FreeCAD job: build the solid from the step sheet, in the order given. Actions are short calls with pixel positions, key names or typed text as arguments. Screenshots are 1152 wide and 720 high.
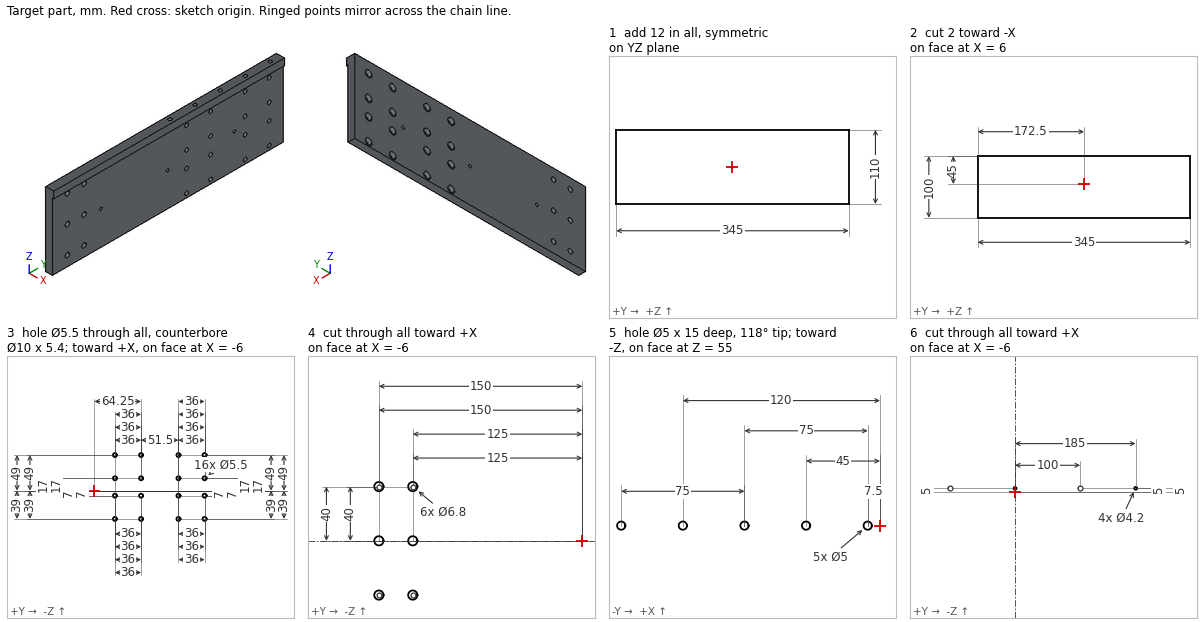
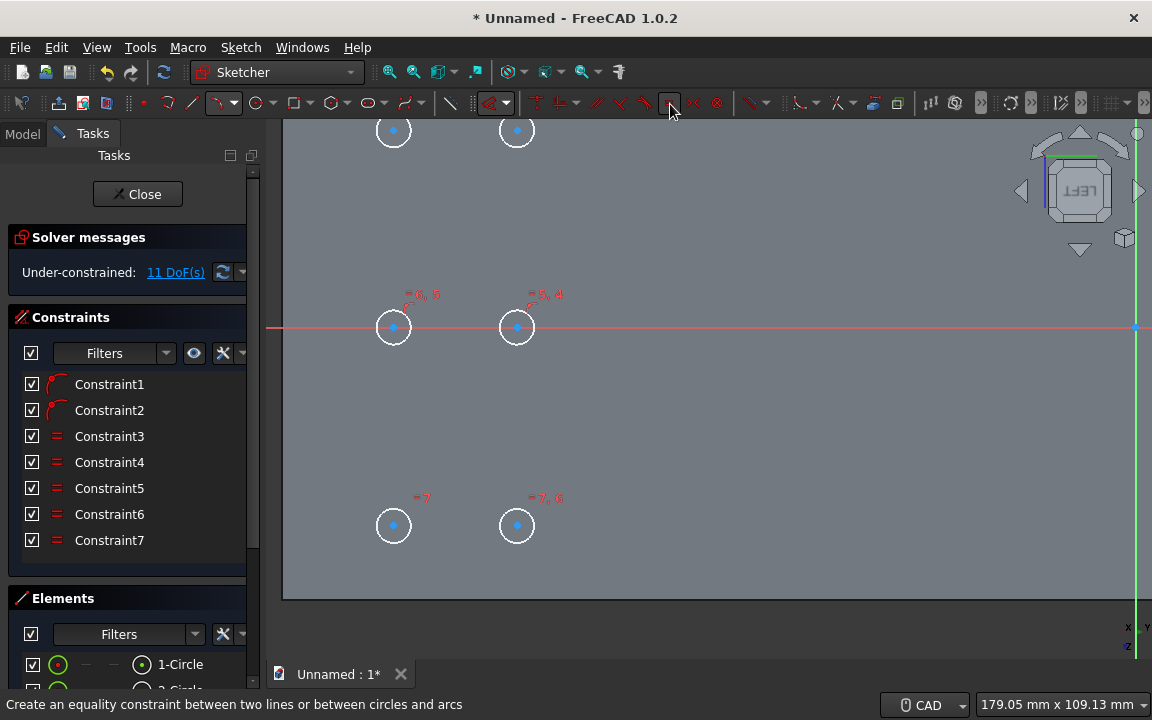
scroll(405, 514, down, 2)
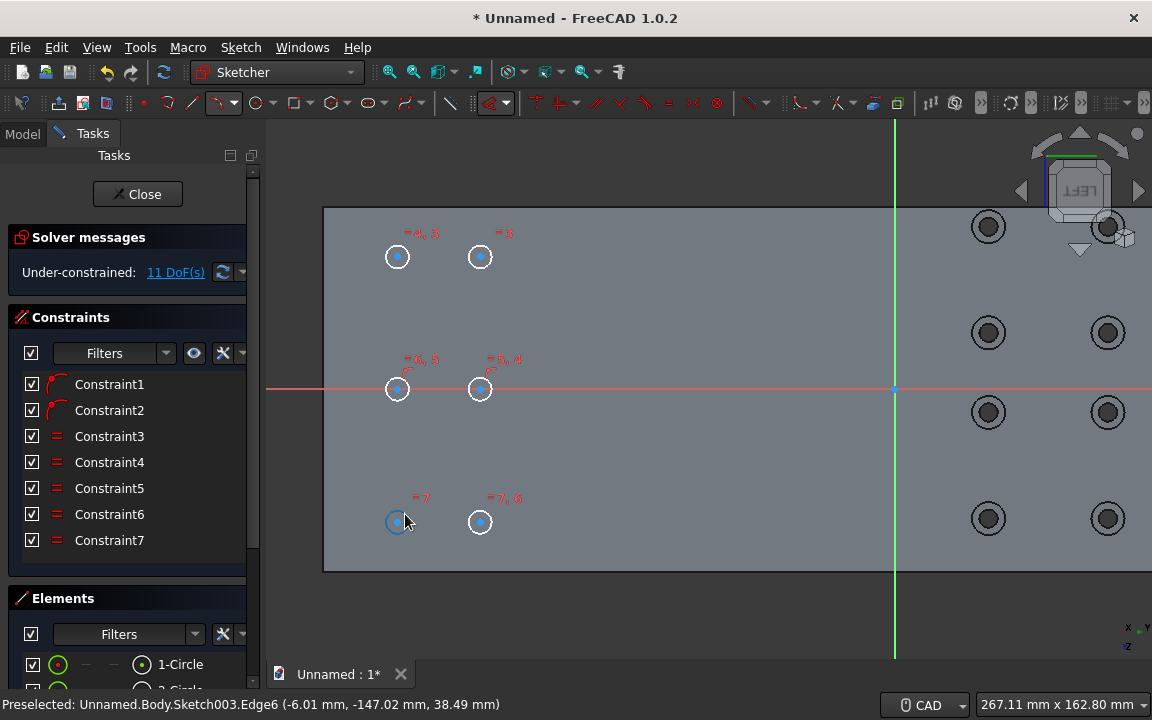
click(480, 257)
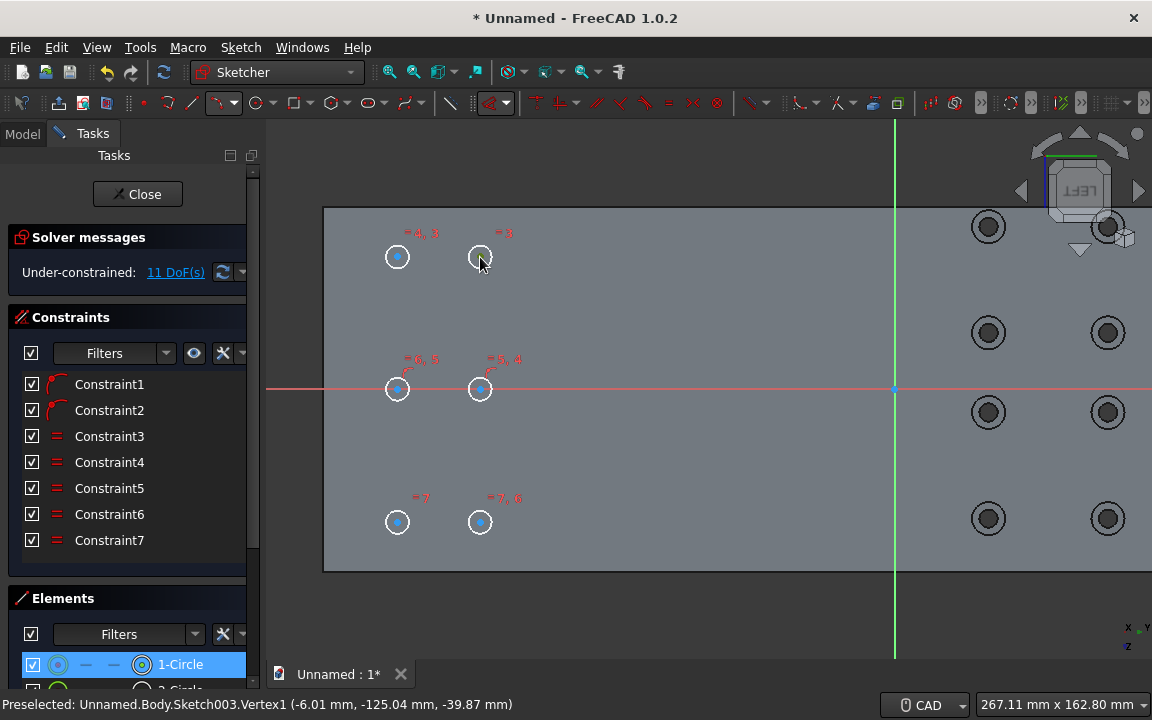
click(480, 522)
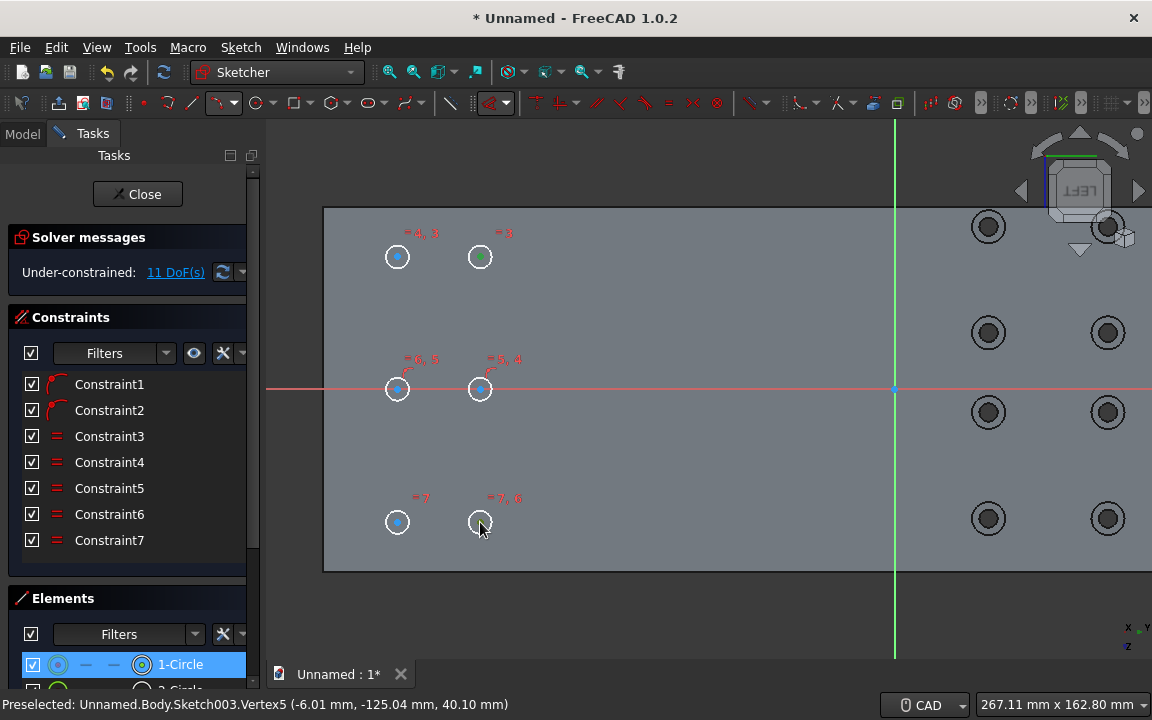
click(344, 389)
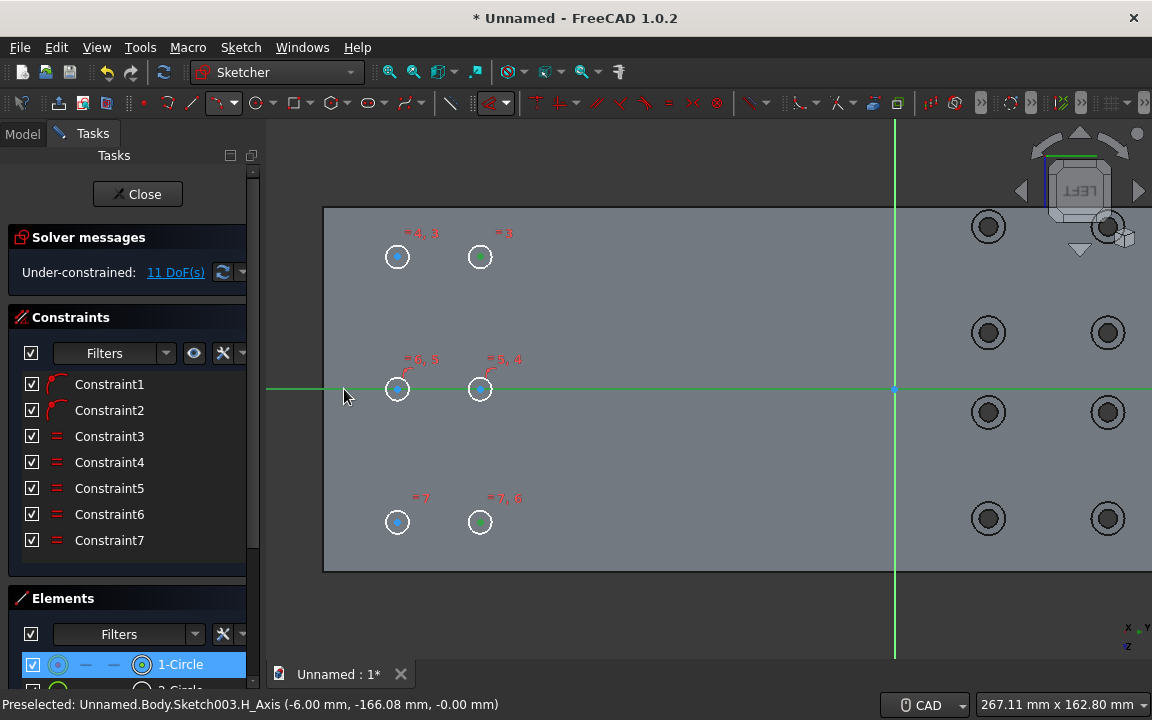
click(694, 104)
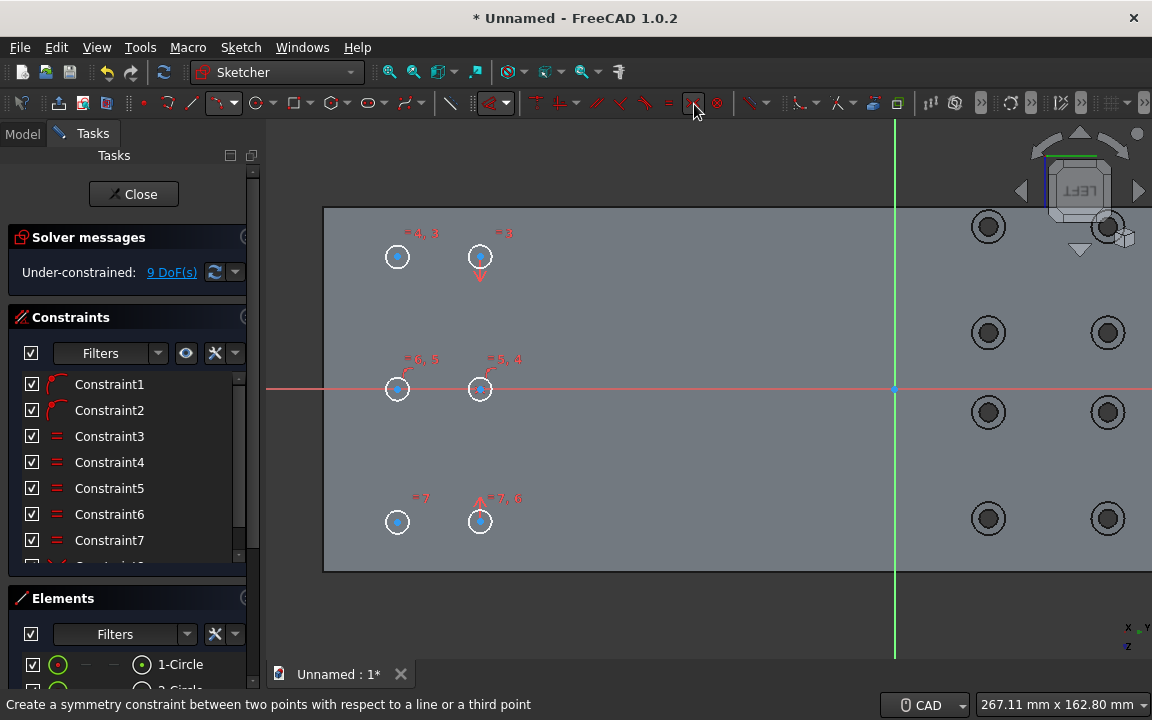
click(397, 257)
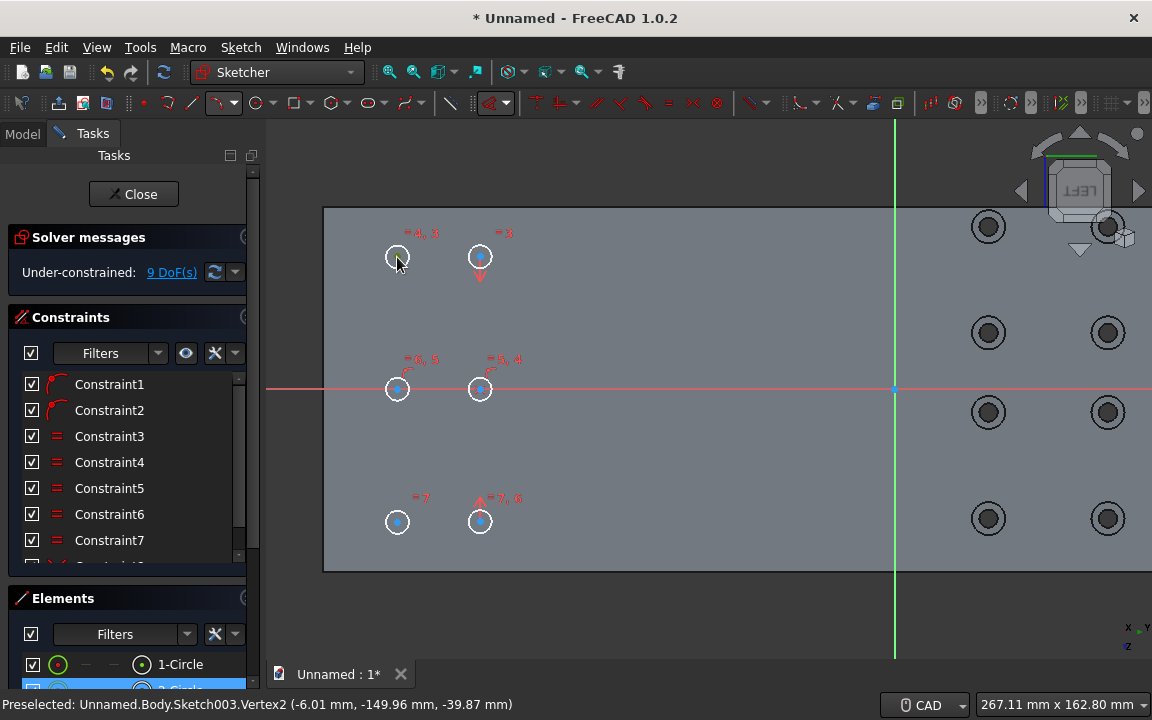
click(397, 522)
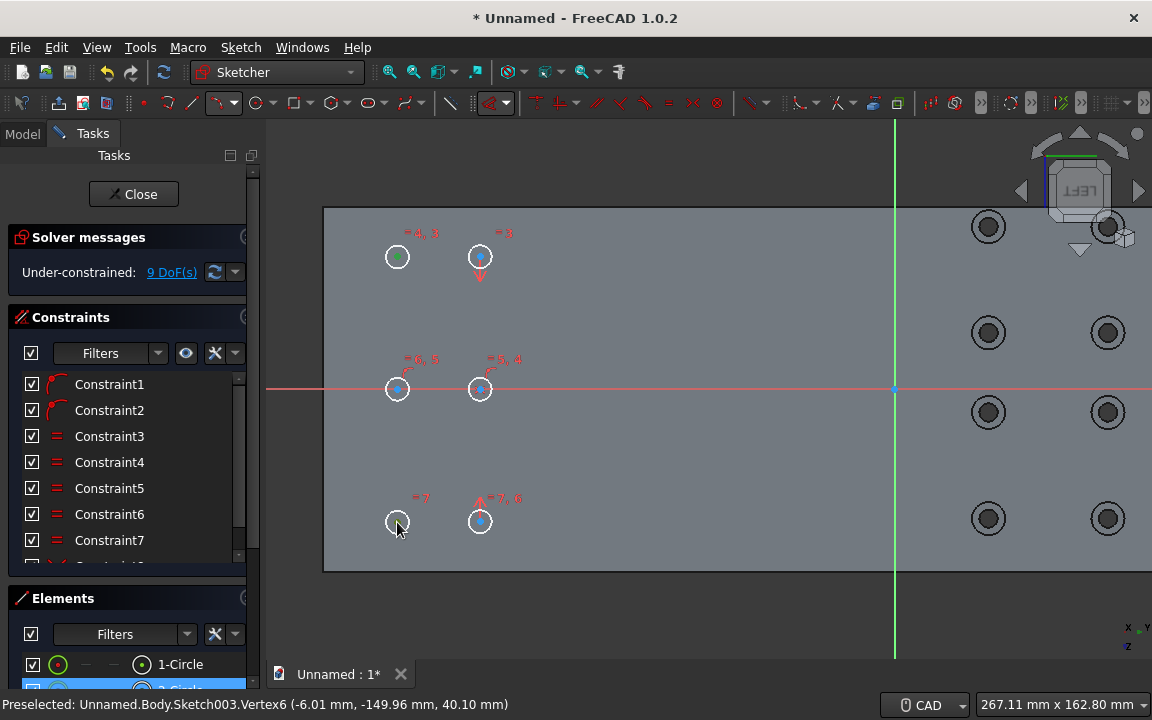
click(344, 389)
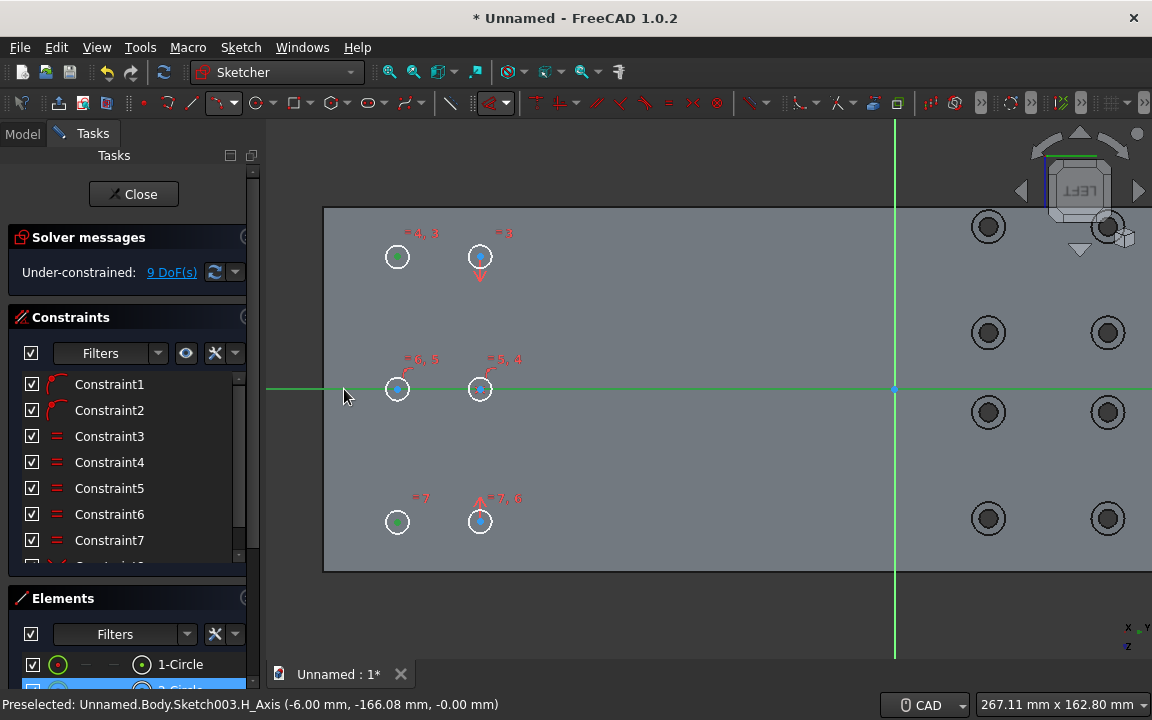
click(694, 104)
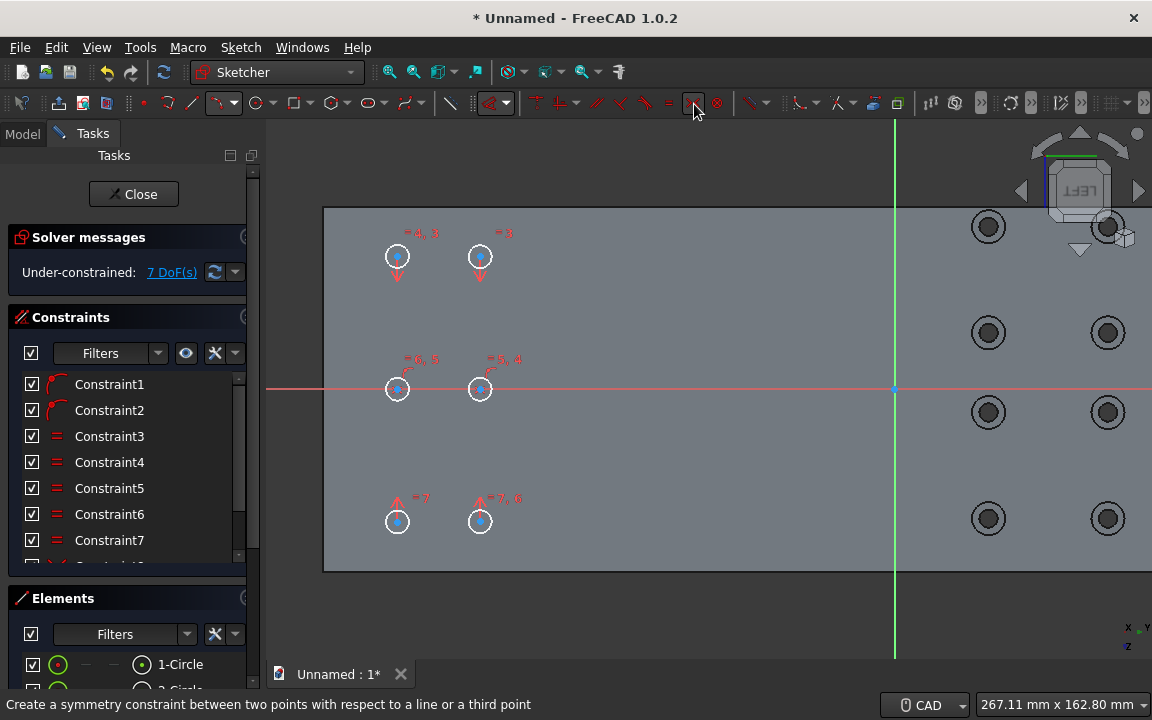
scroll(488, 249, up, 3)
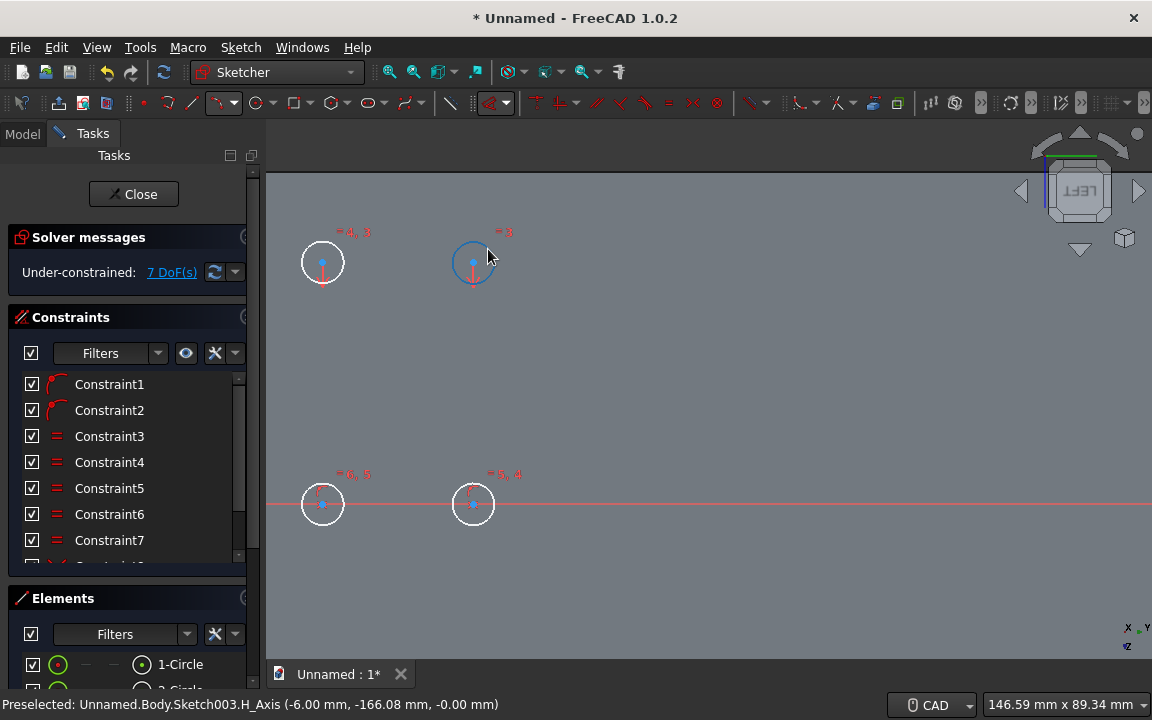
click(488, 248)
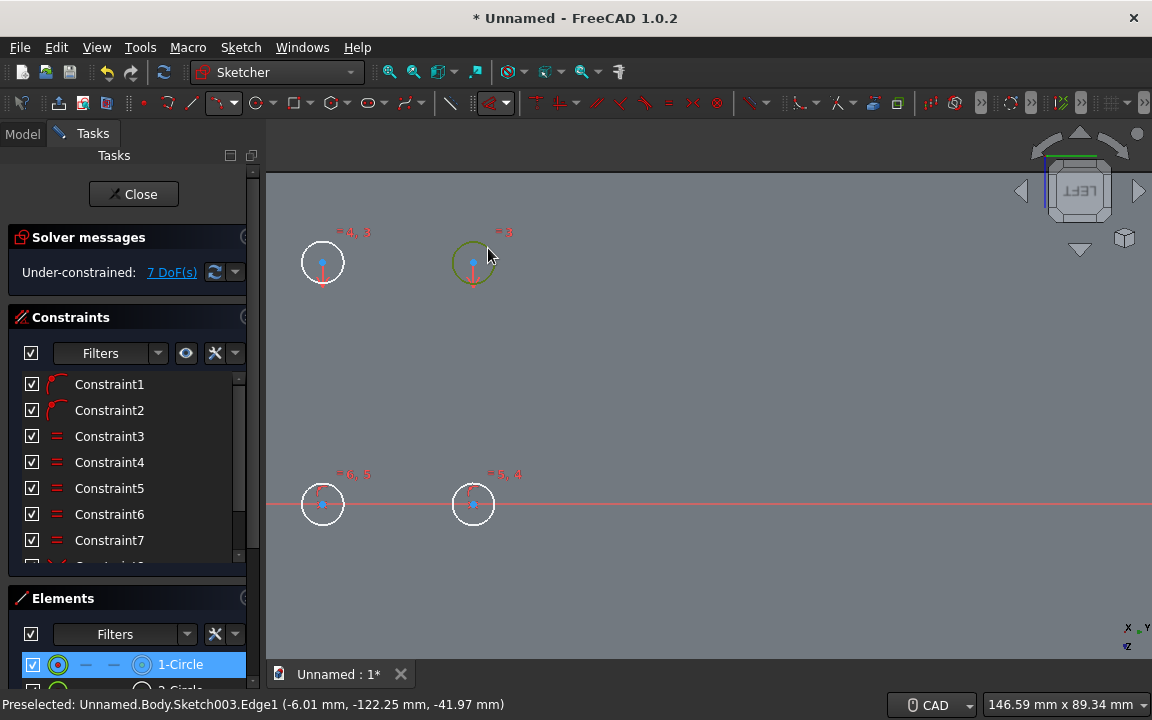
key(k)
key(o)